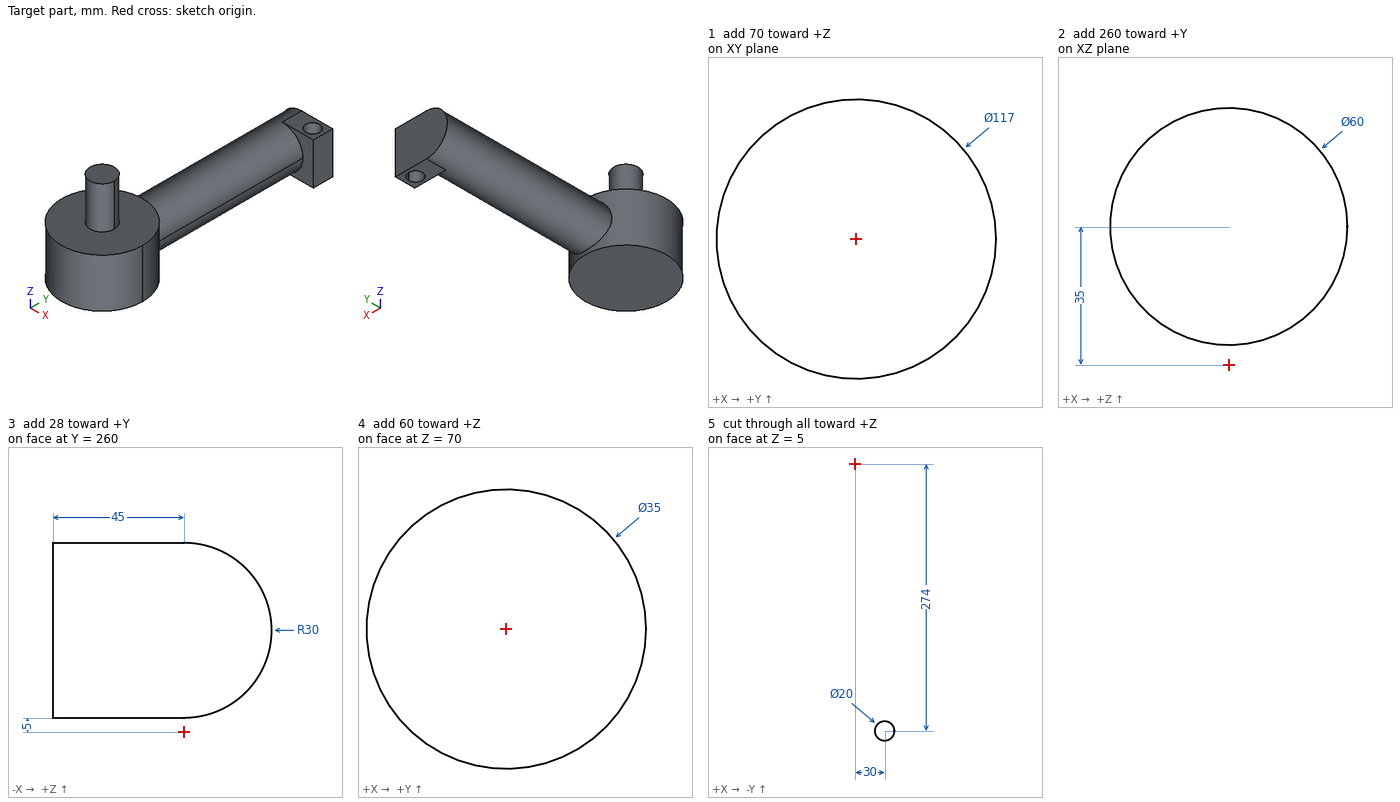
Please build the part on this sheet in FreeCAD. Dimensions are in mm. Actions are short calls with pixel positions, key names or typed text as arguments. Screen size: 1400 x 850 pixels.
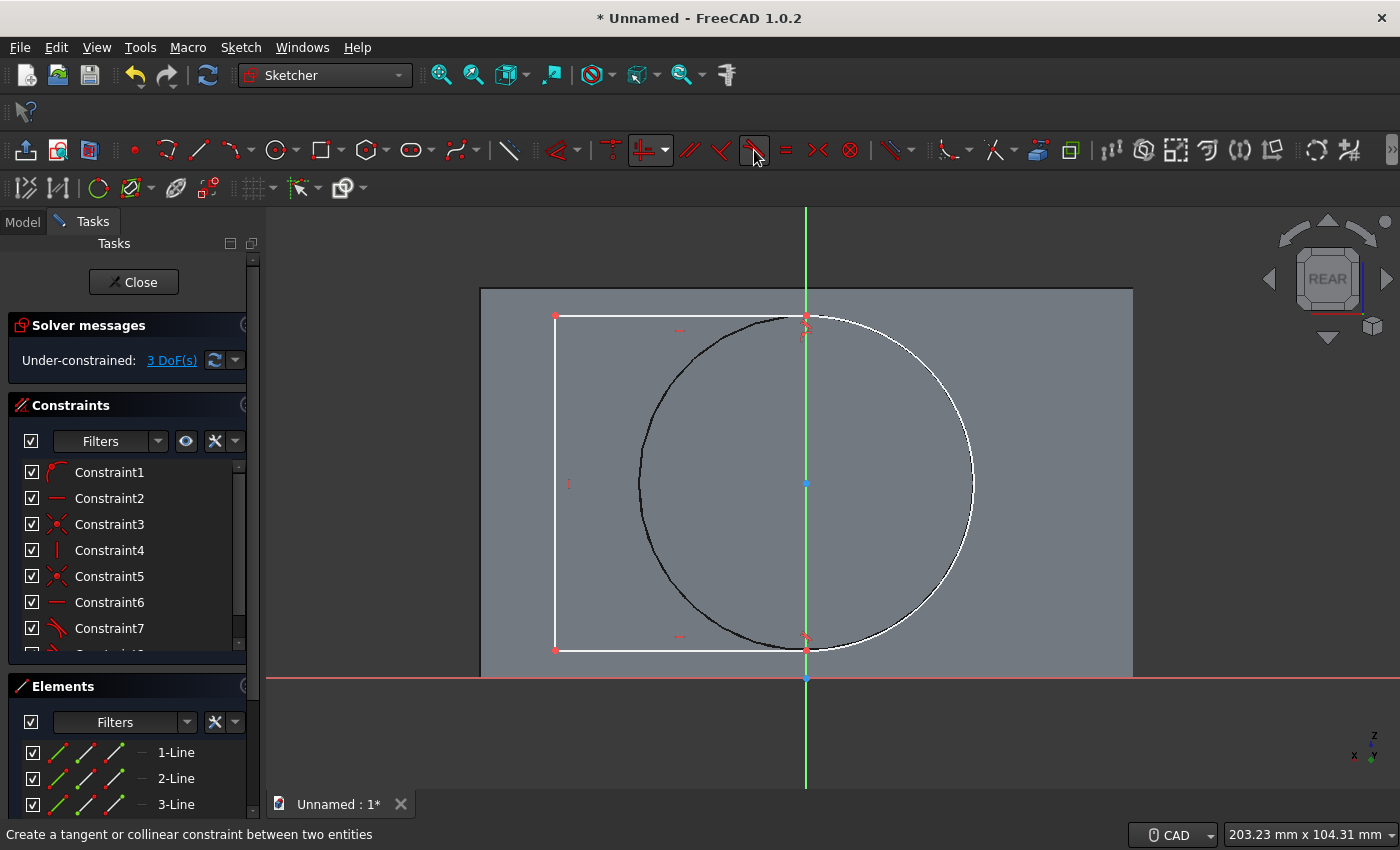
key(d)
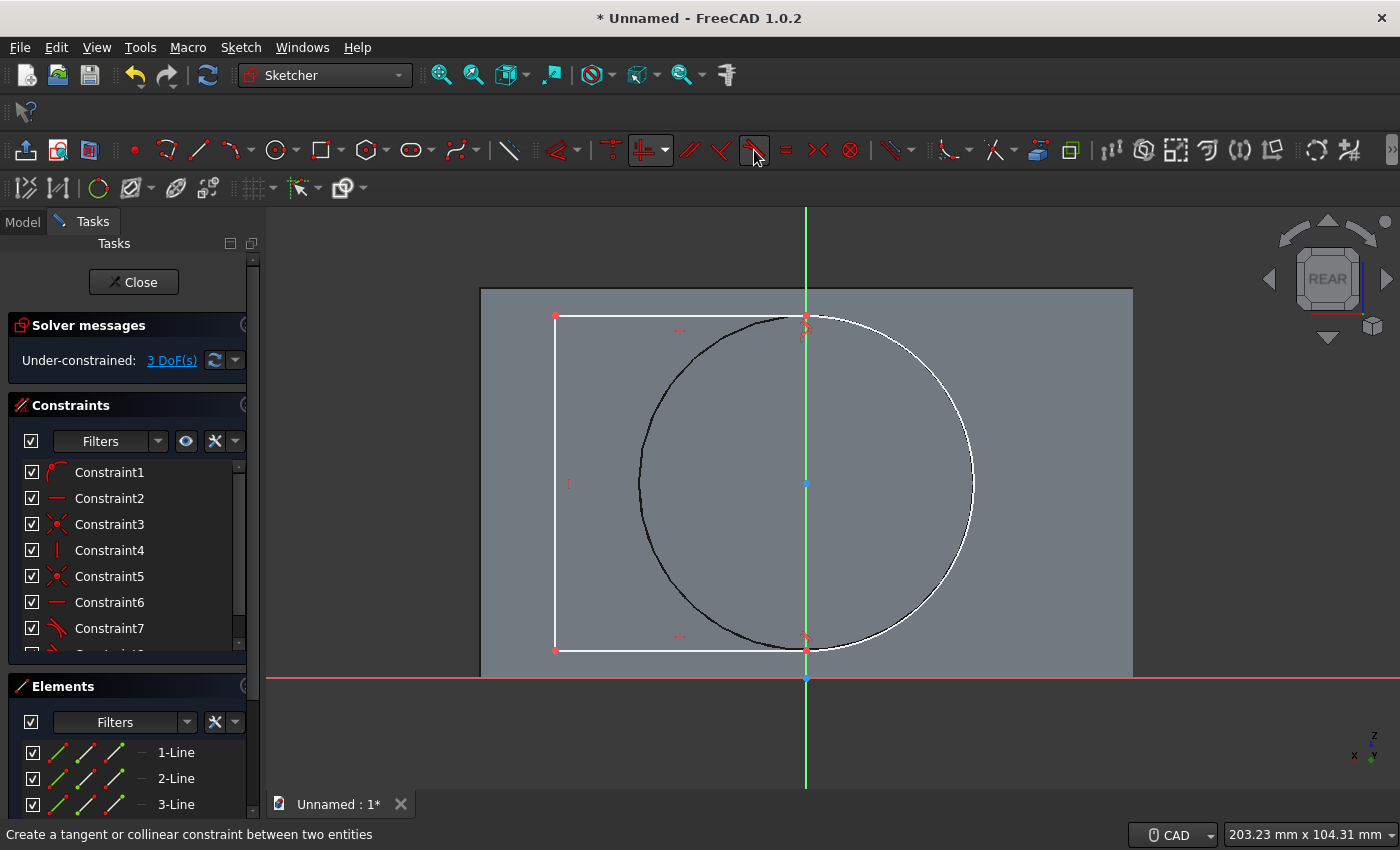
click(942, 582)
click(968, 601)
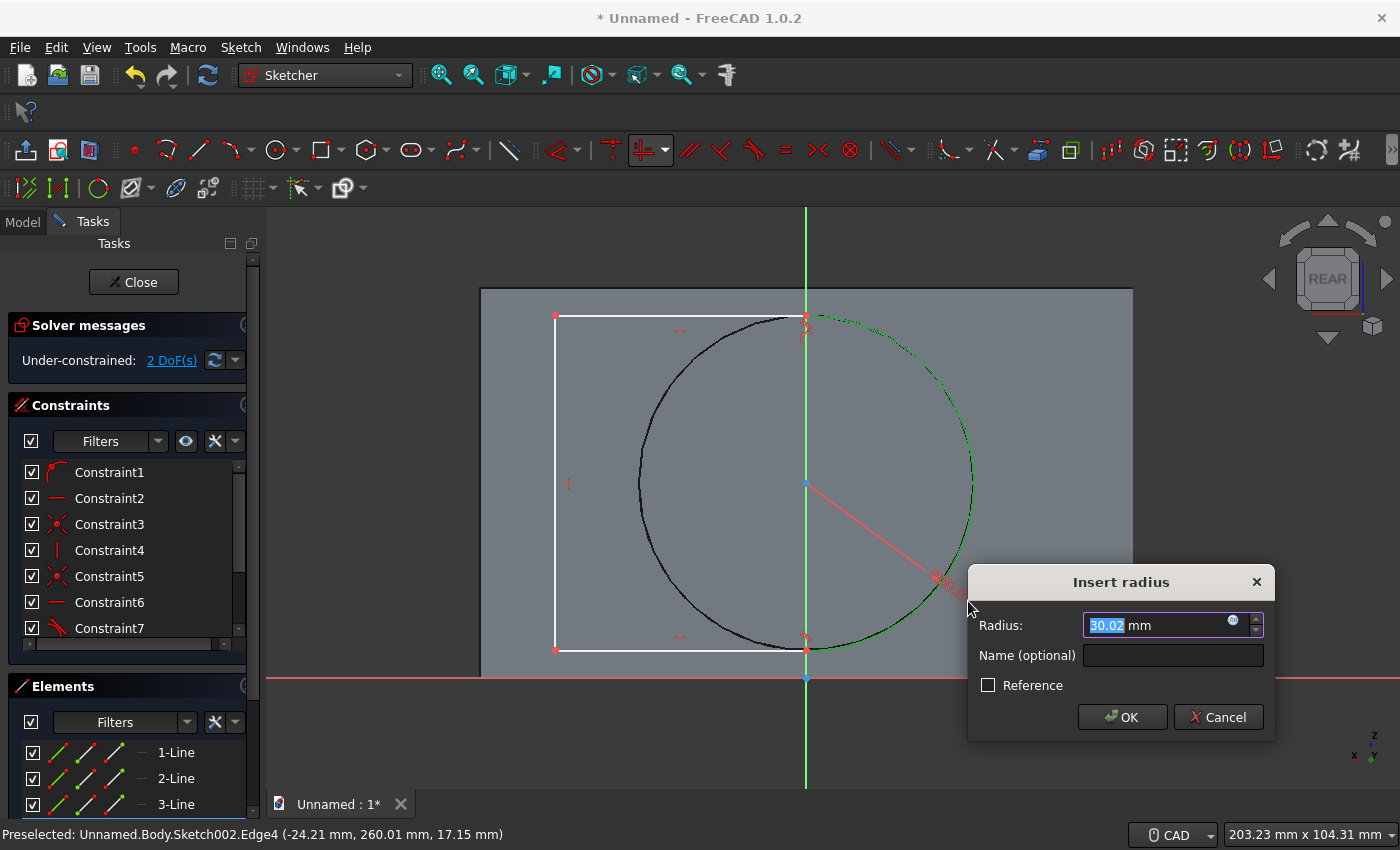
text(30)
key(Return)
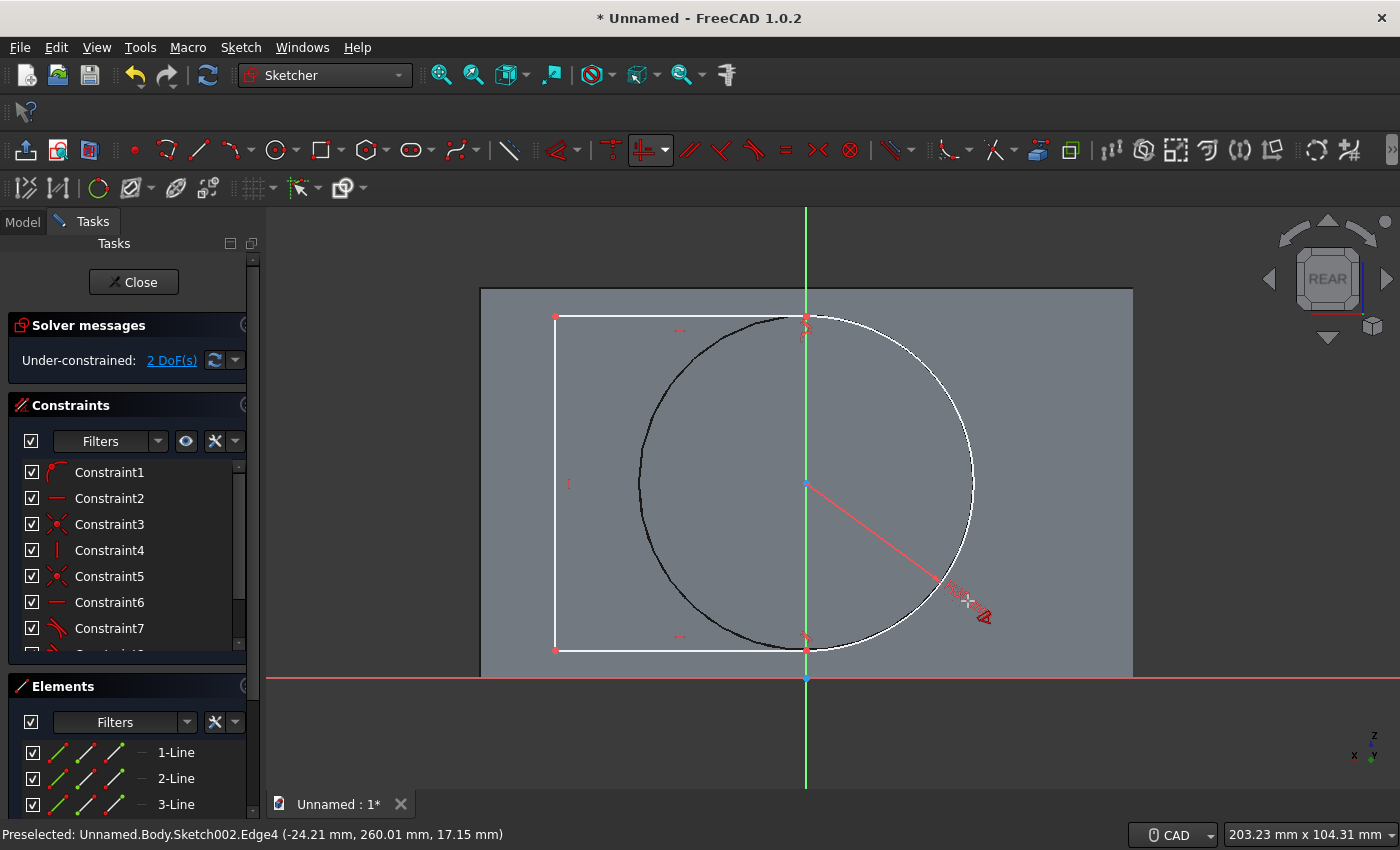
click(731, 316)
click(681, 282)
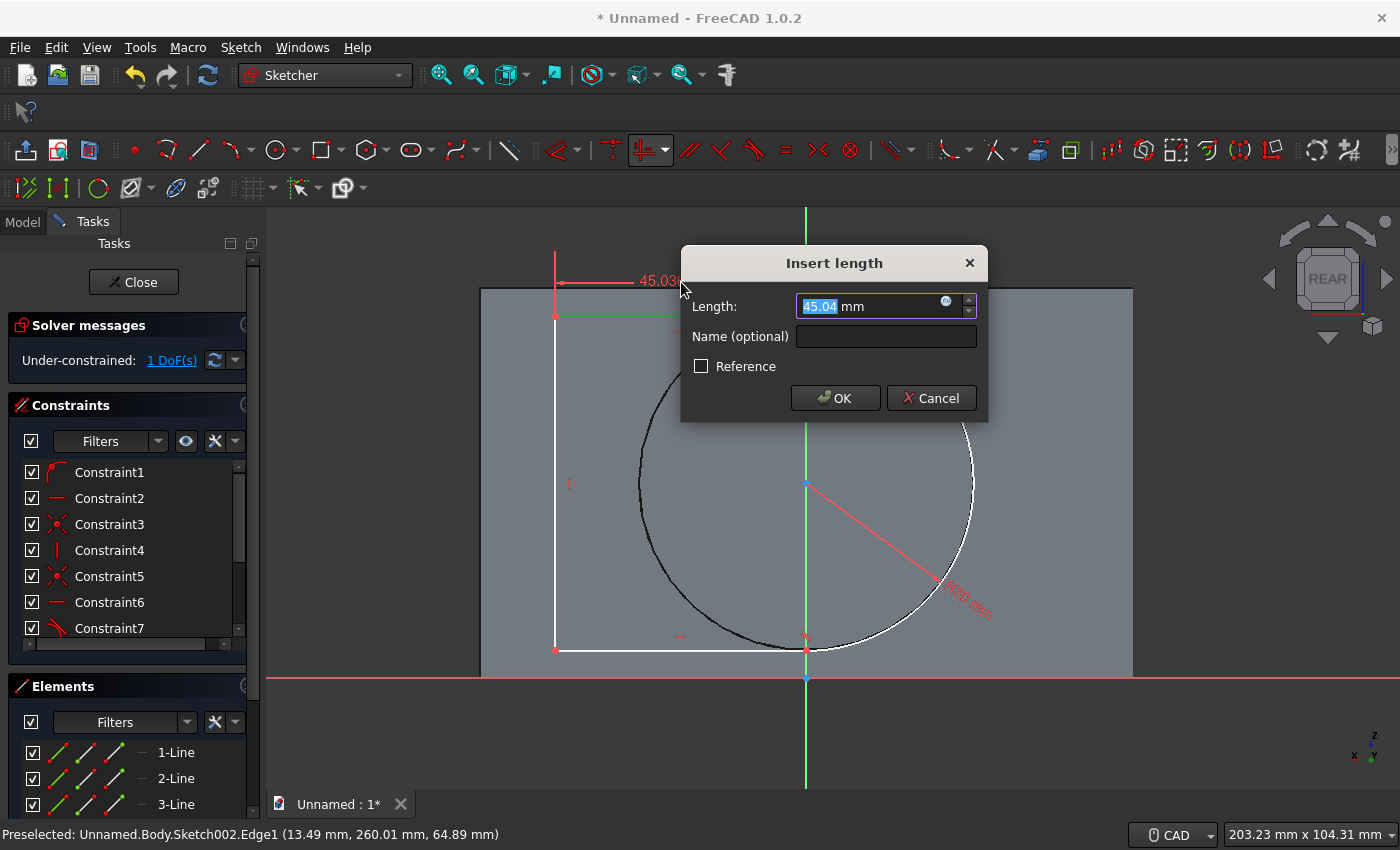
text(45)
key(Return)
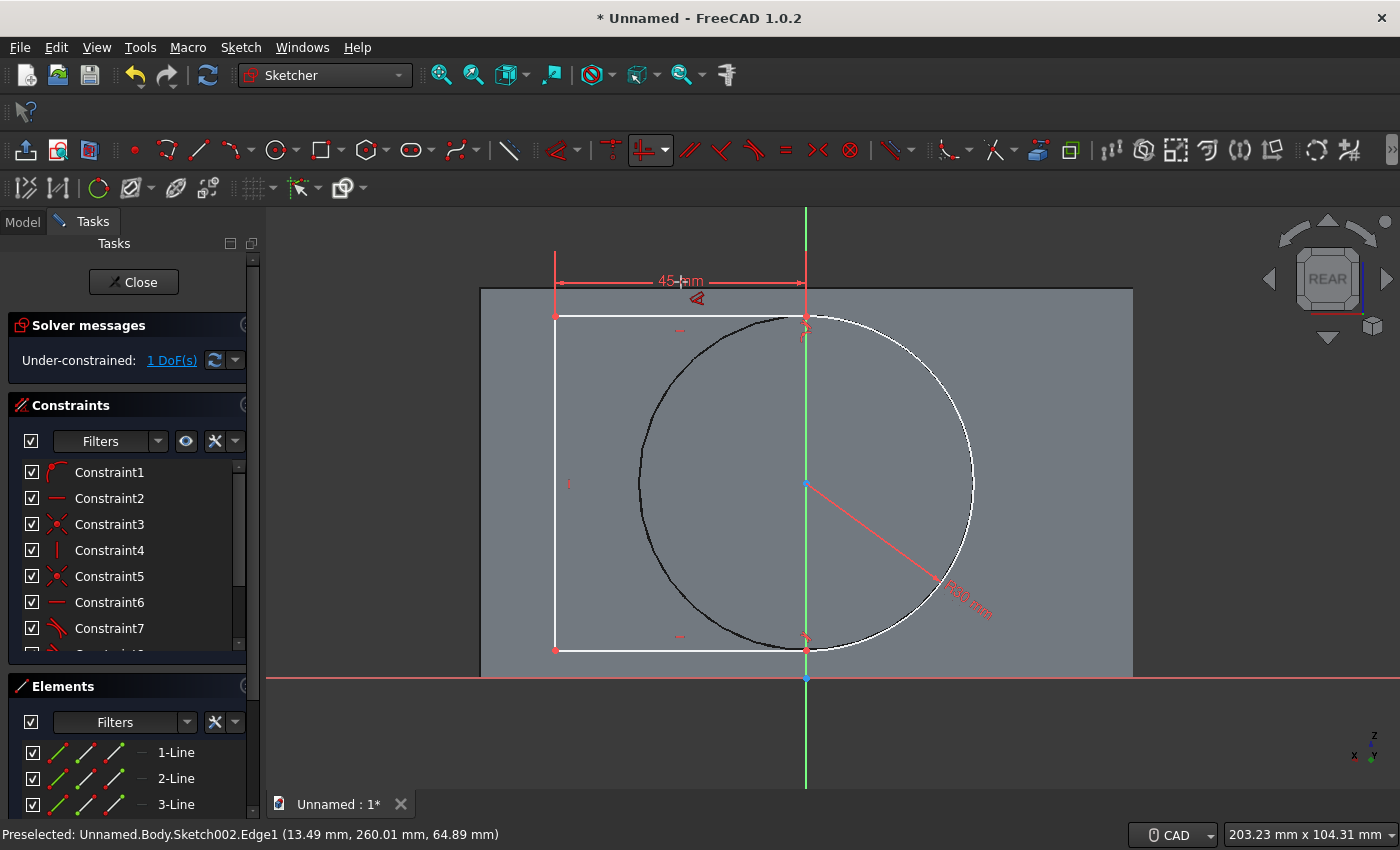
scroll(555, 651, up, 2)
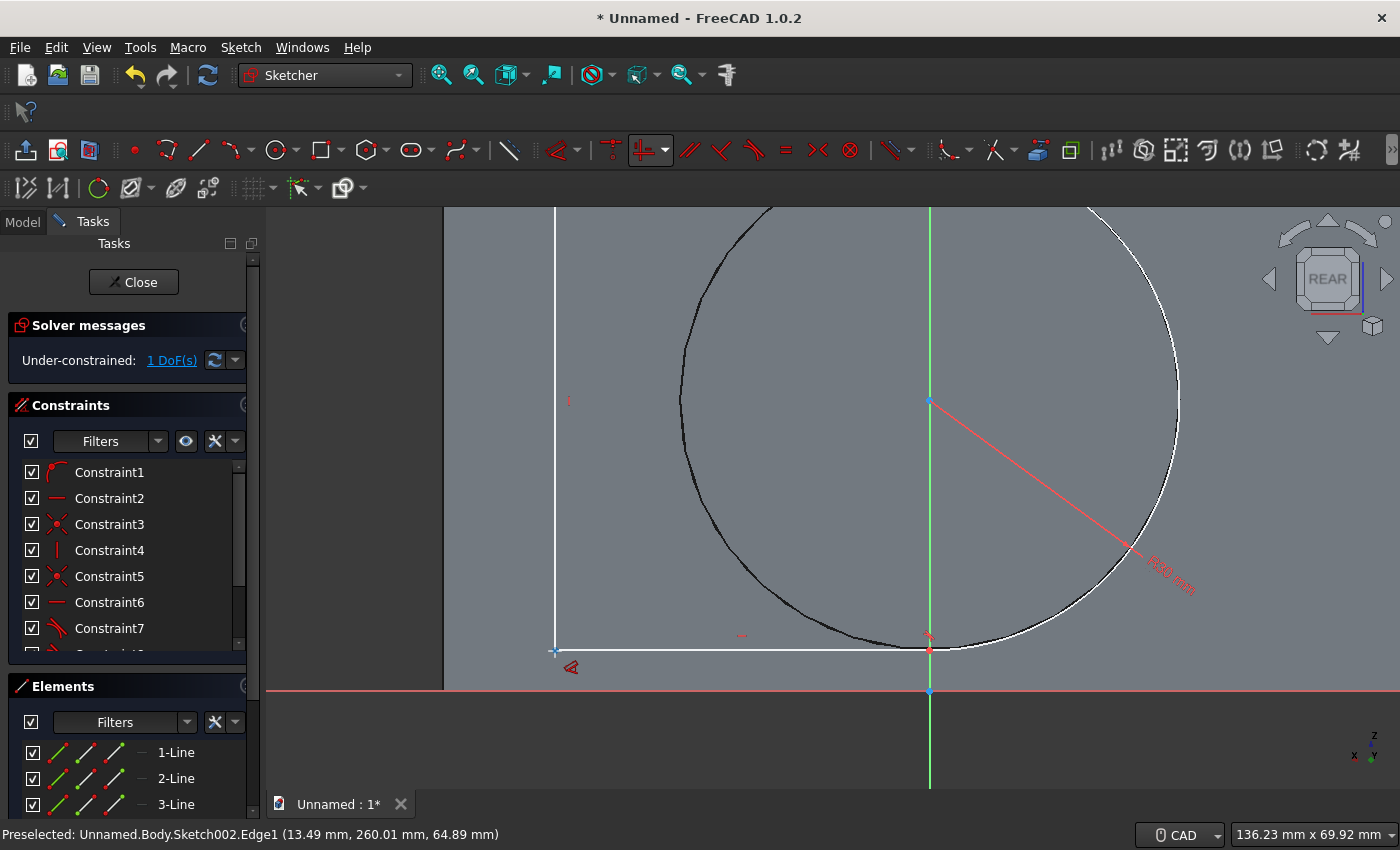
click(555, 650)
click(521, 671)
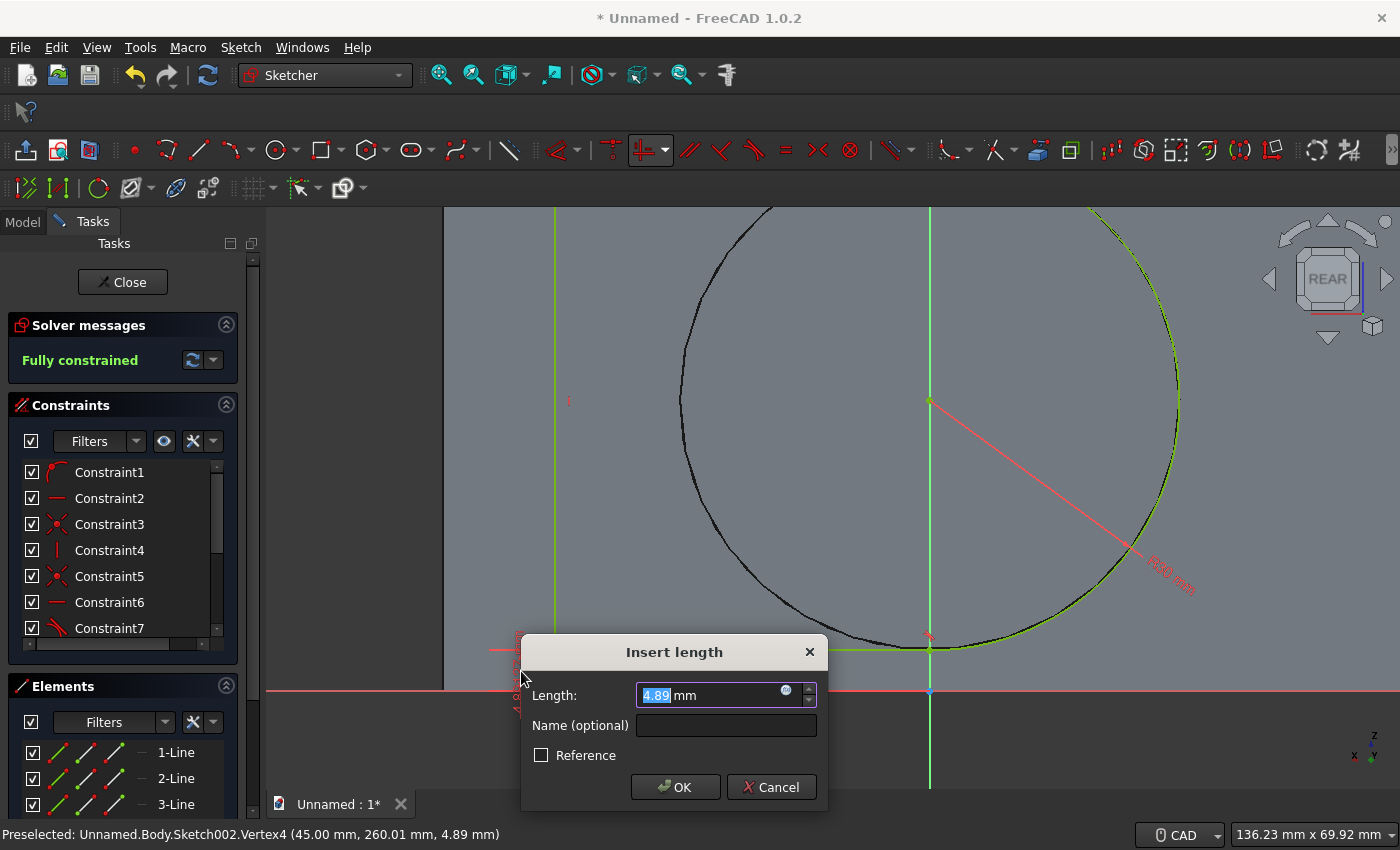
text(5)
key(Return)
key(Escape)